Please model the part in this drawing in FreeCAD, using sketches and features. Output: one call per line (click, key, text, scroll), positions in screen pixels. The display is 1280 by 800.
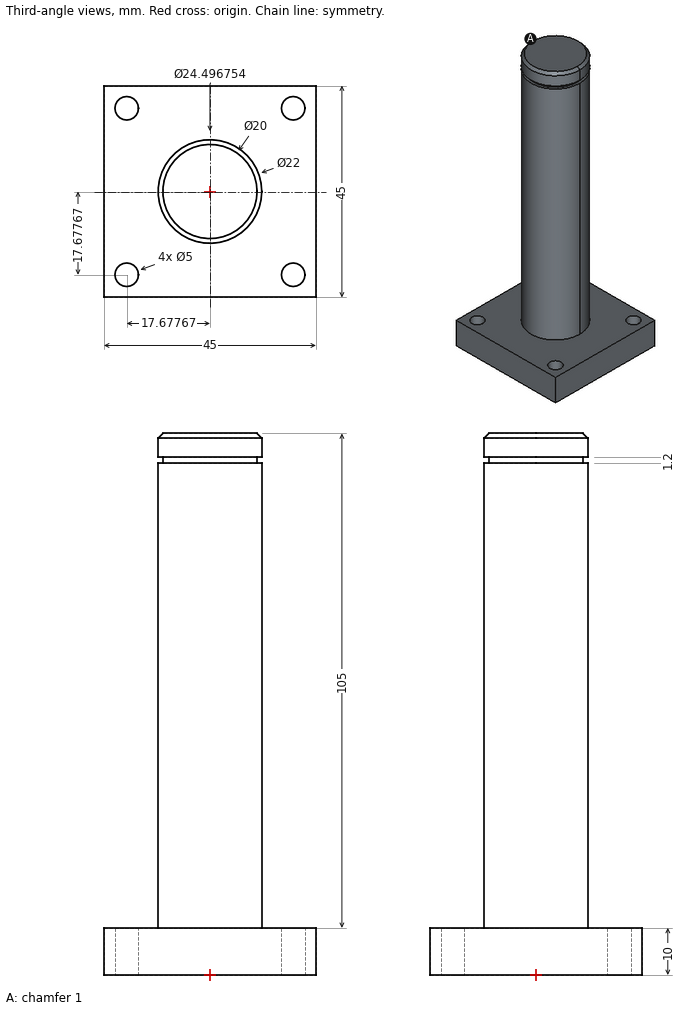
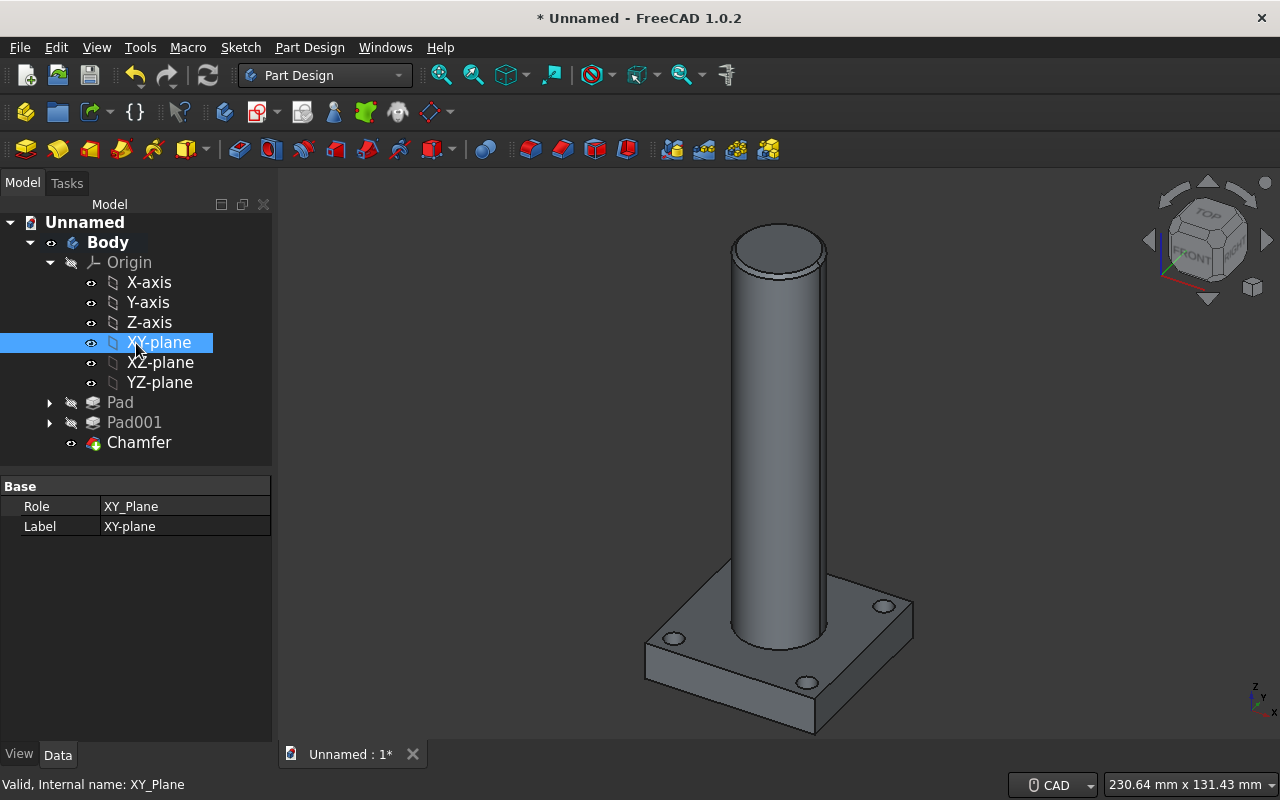
click(430, 112)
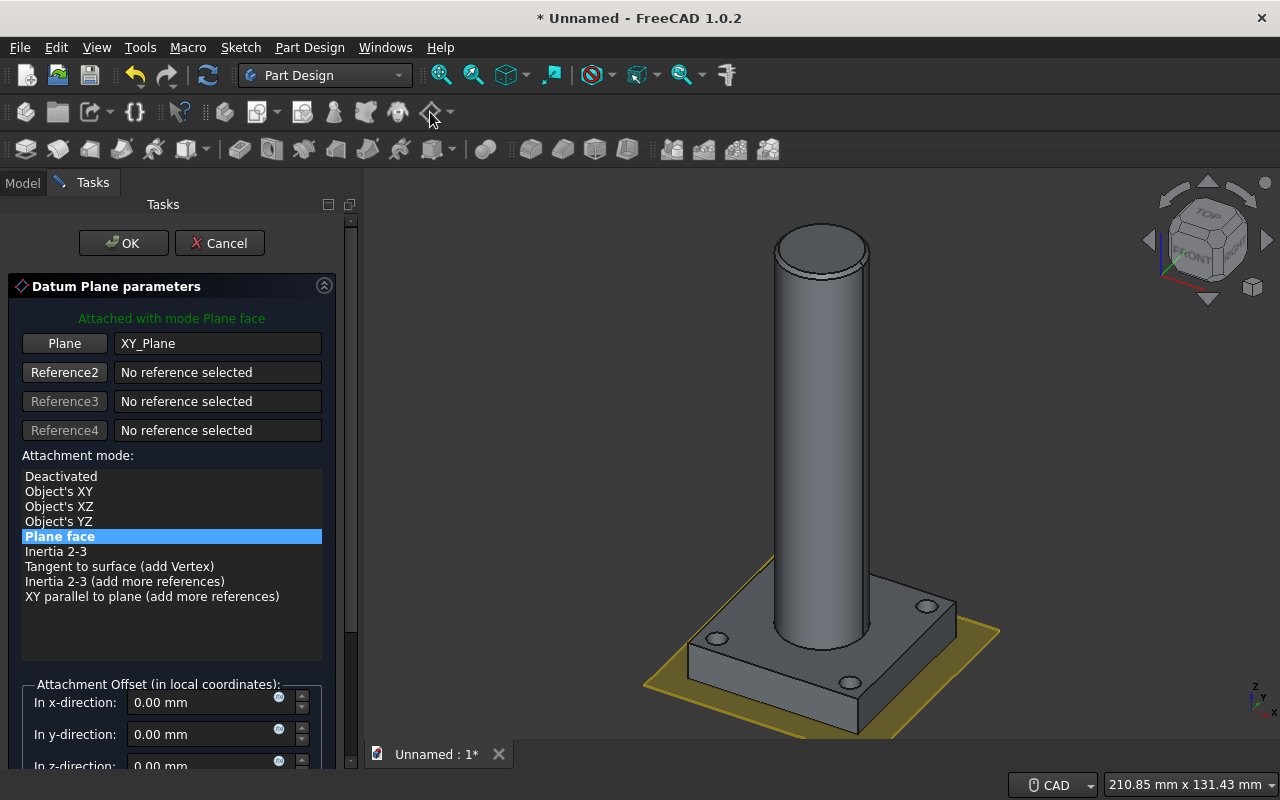
scroll(351, 491, down, 2)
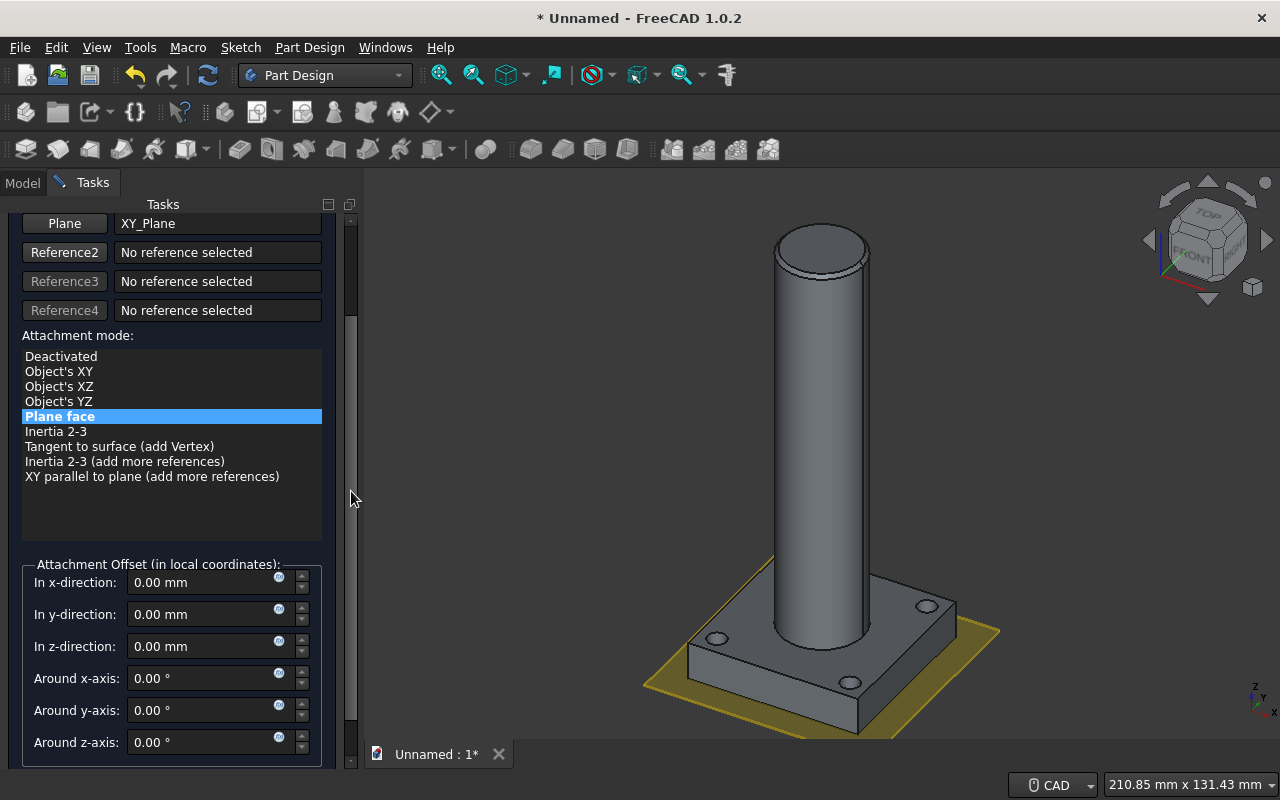
triple_click(210, 646)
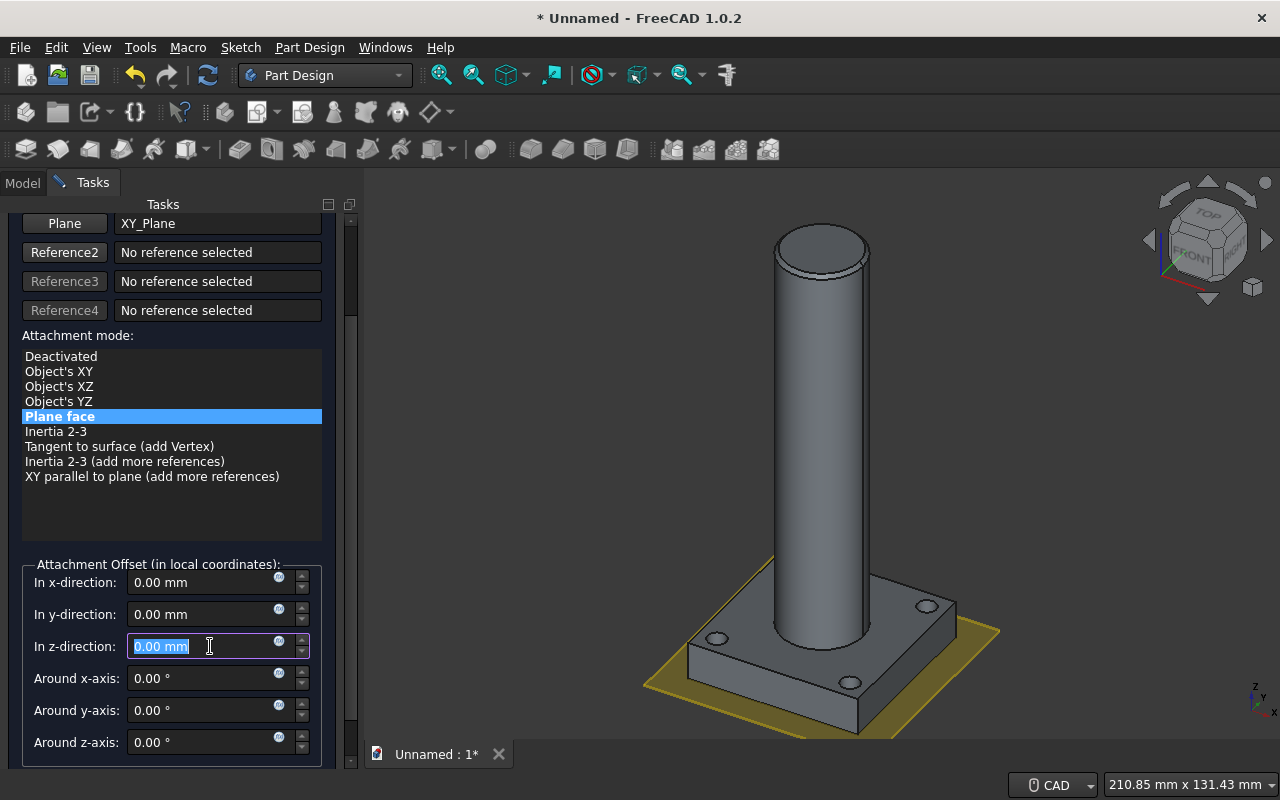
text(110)
key(Tab)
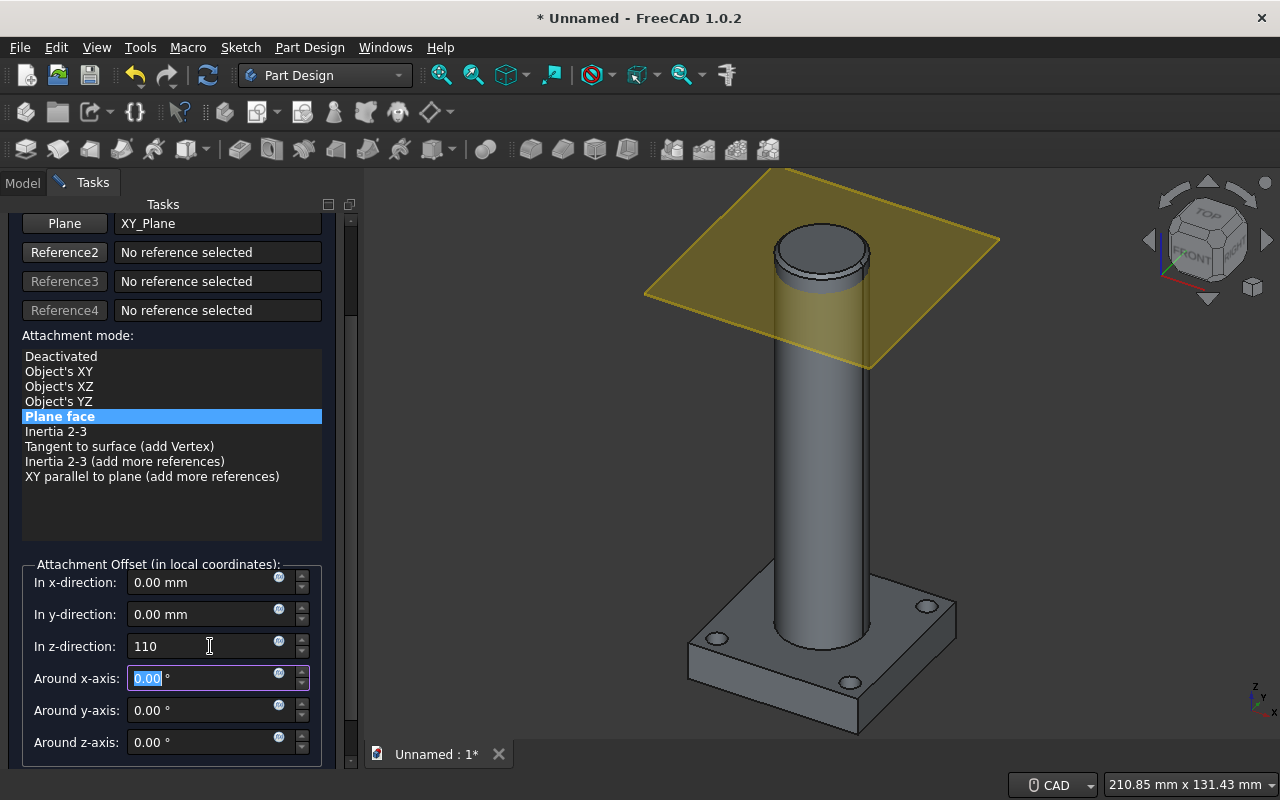
scroll(351, 491, up, 3)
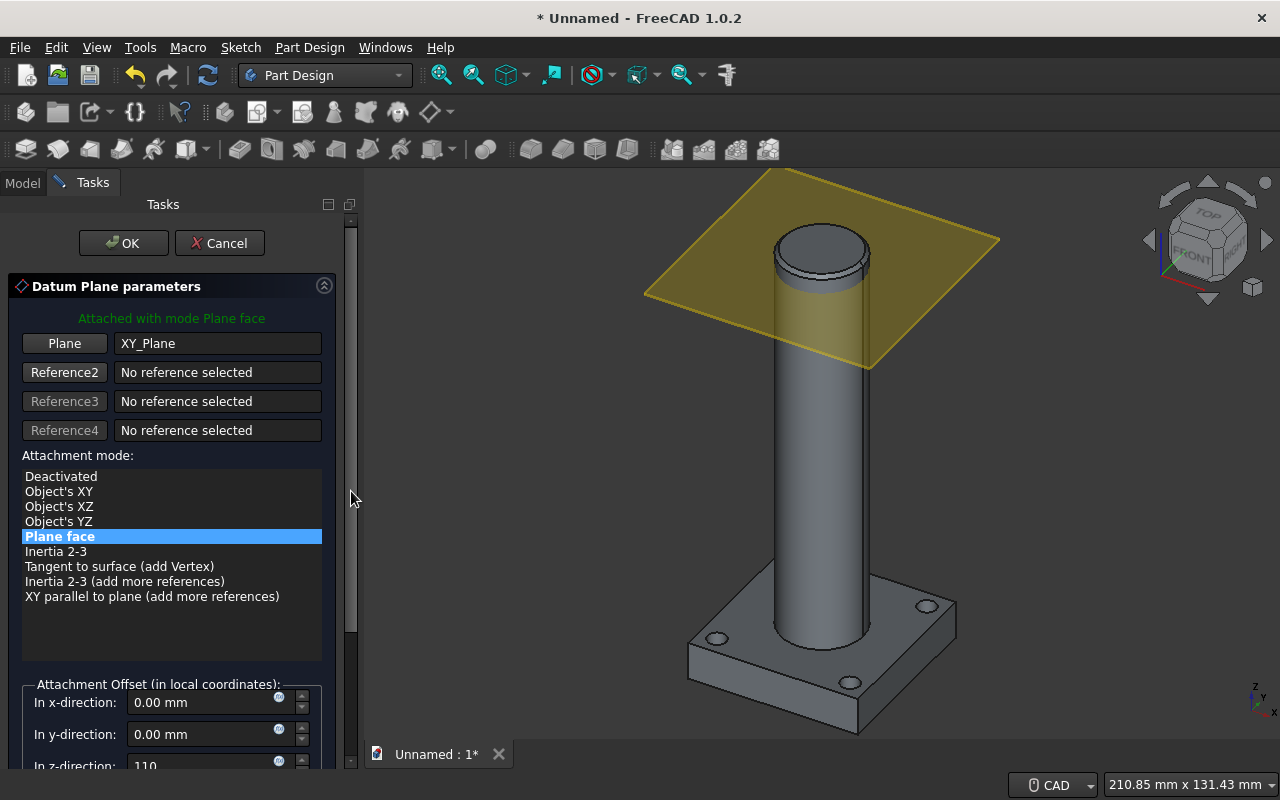
click(124, 243)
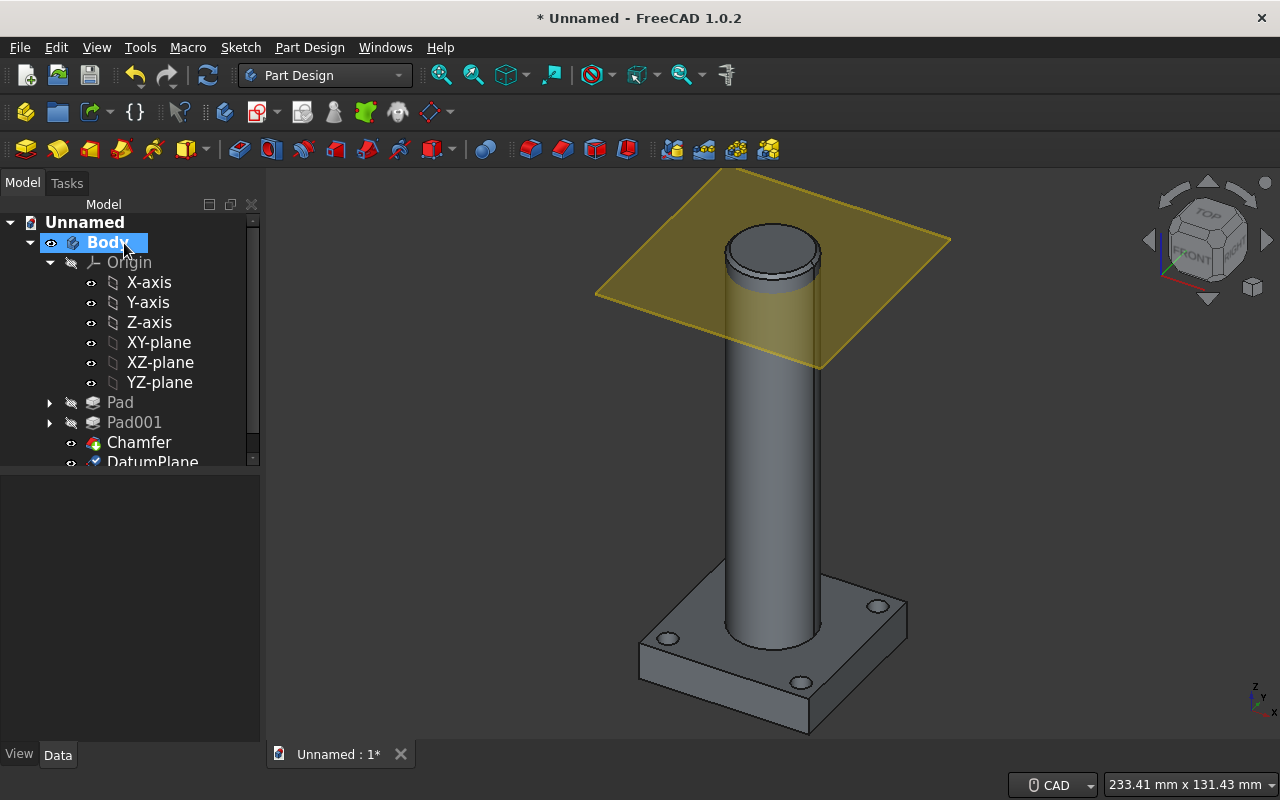
click(116, 463)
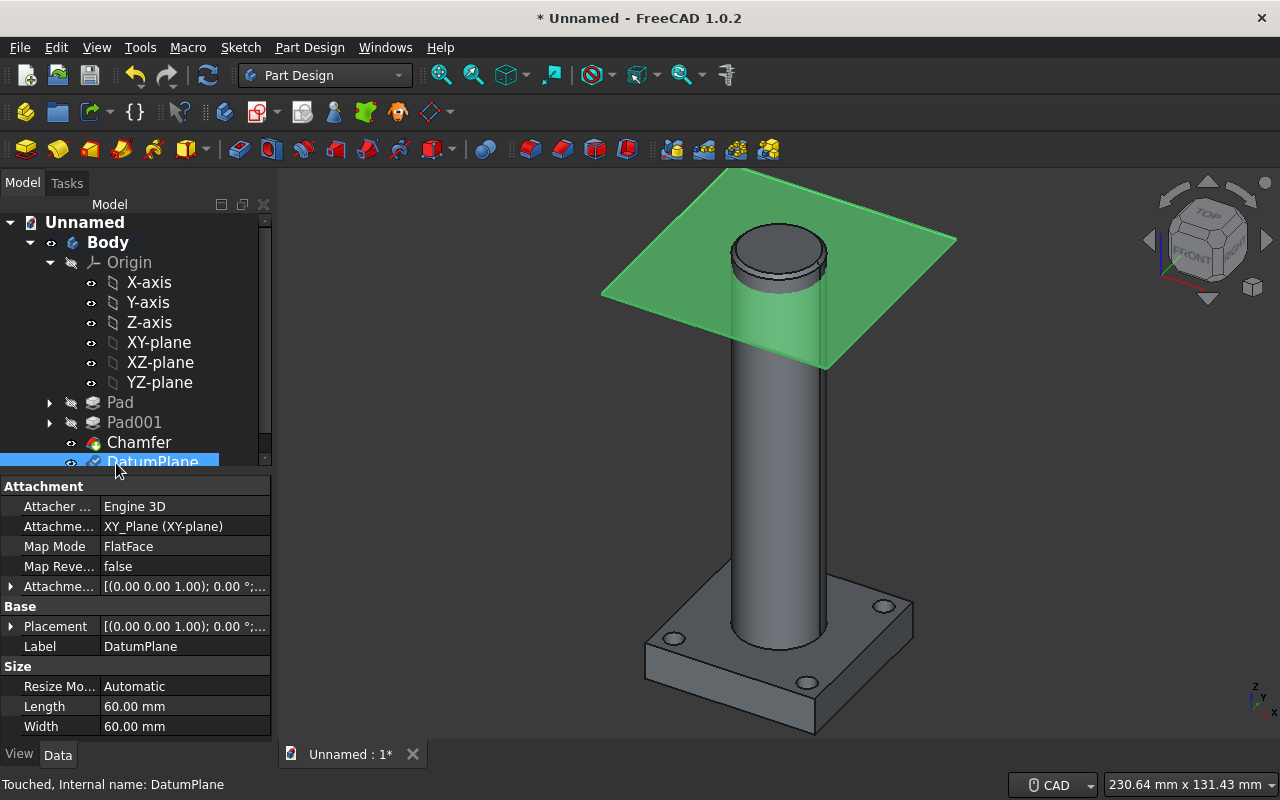
click(258, 112)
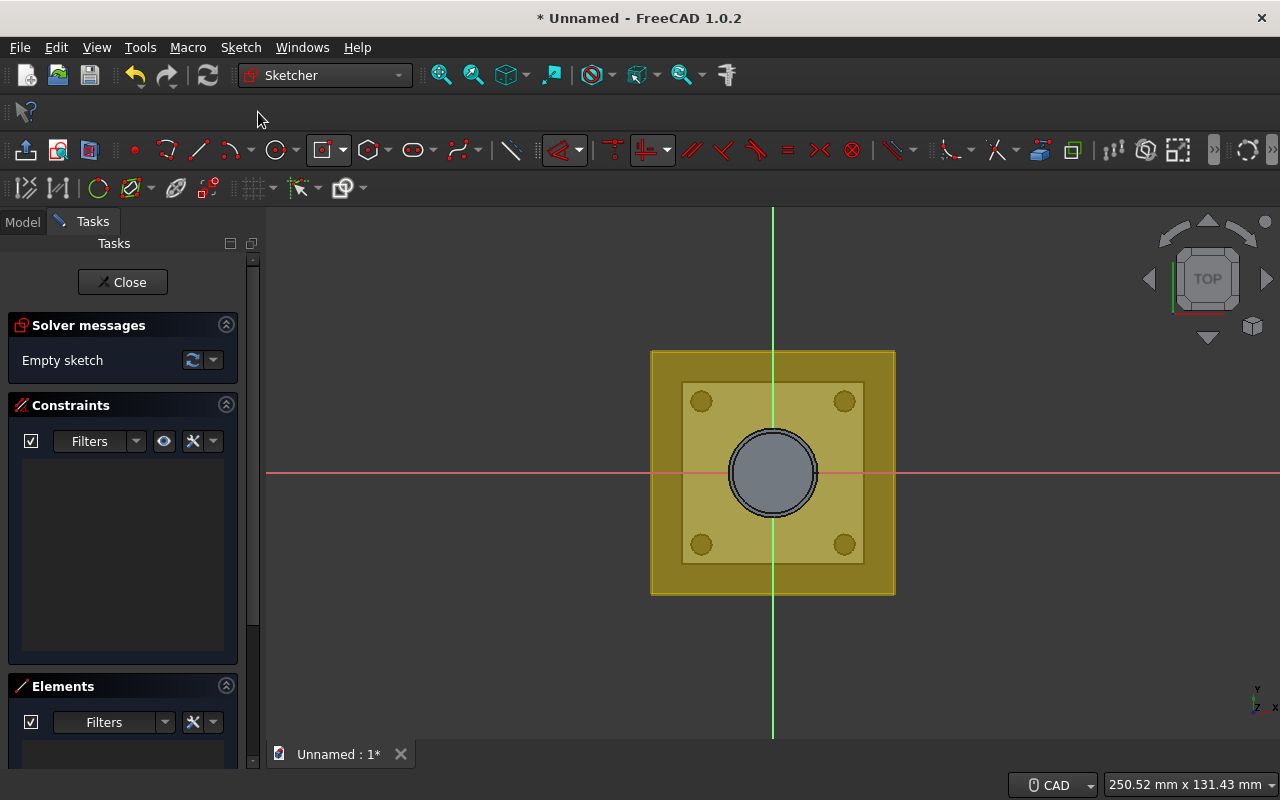
click(90, 150)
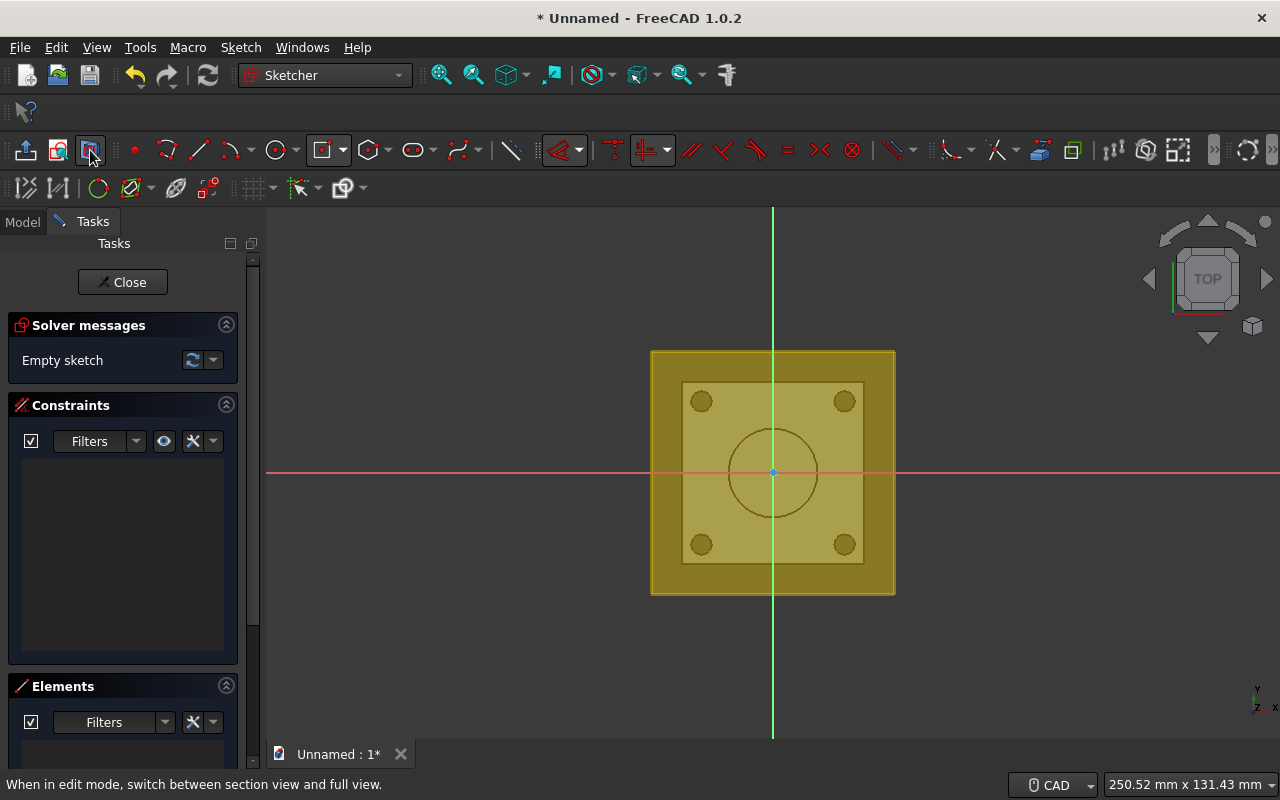
scroll(803, 473, up, 6)